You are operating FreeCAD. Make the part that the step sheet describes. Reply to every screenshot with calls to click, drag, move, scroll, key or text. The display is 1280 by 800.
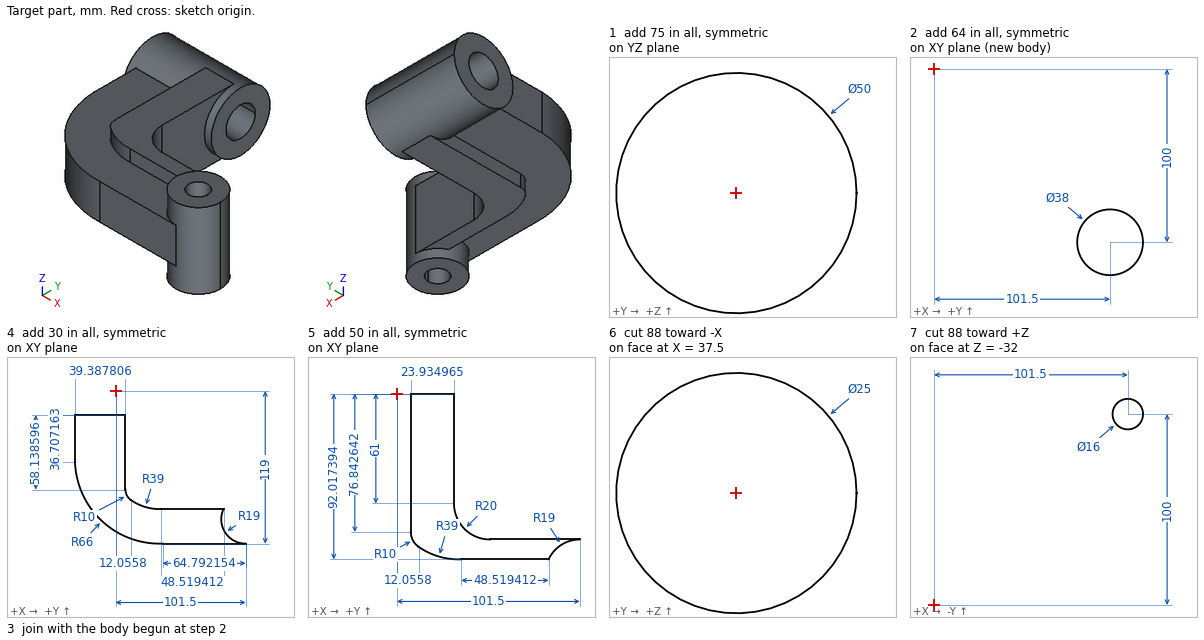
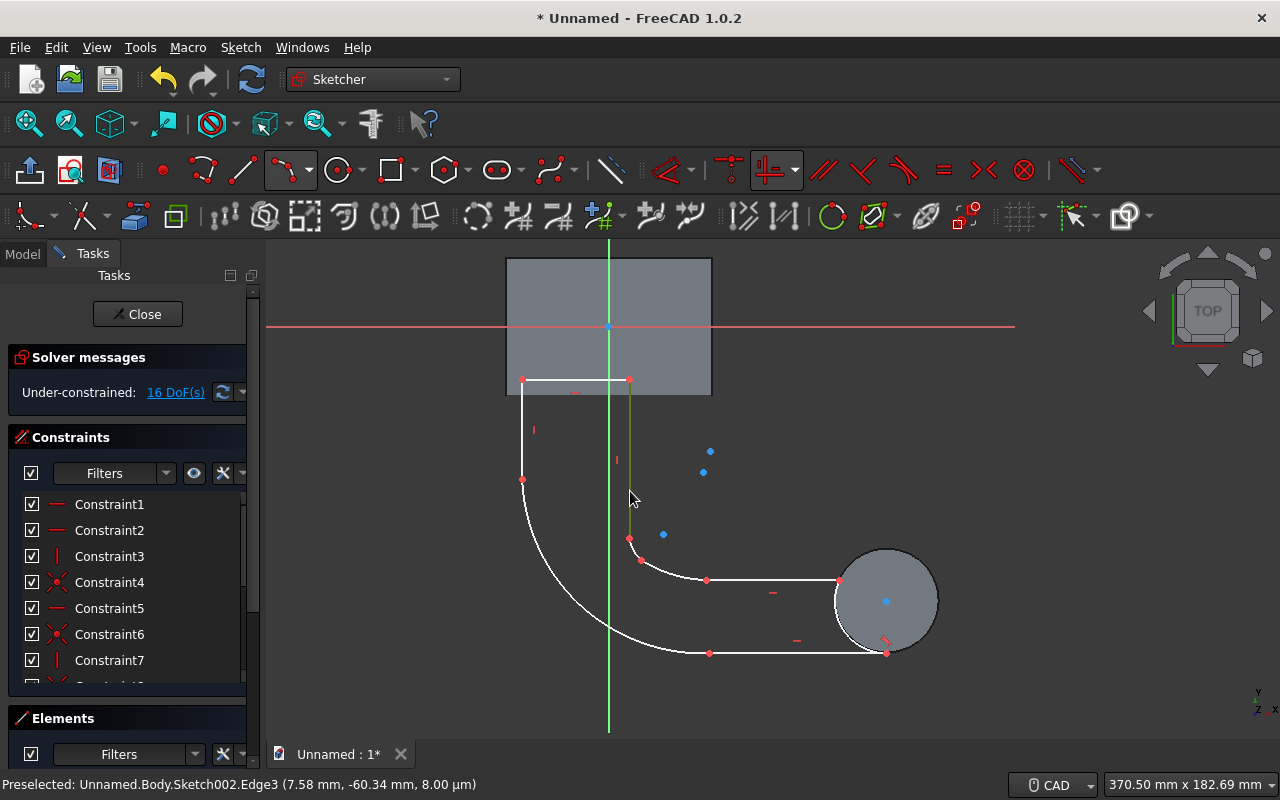
click(634, 551)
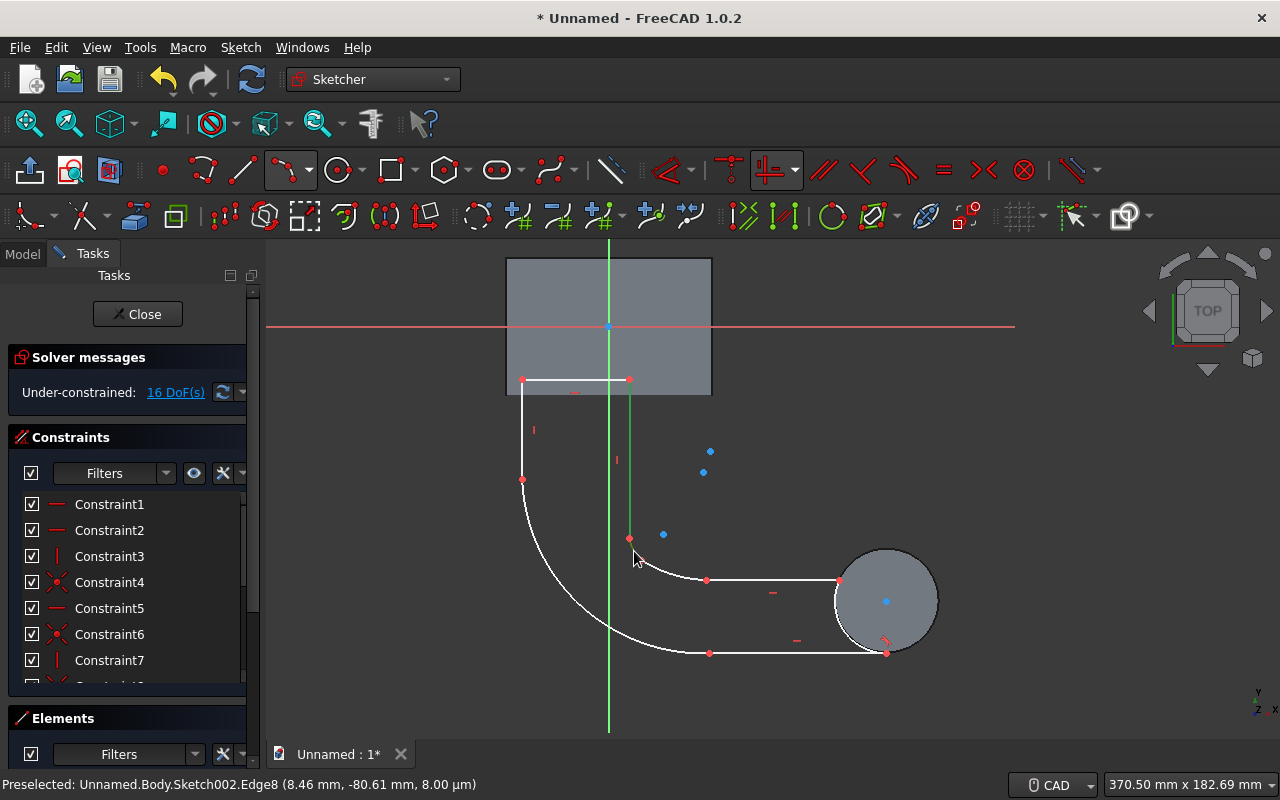
click(904, 170)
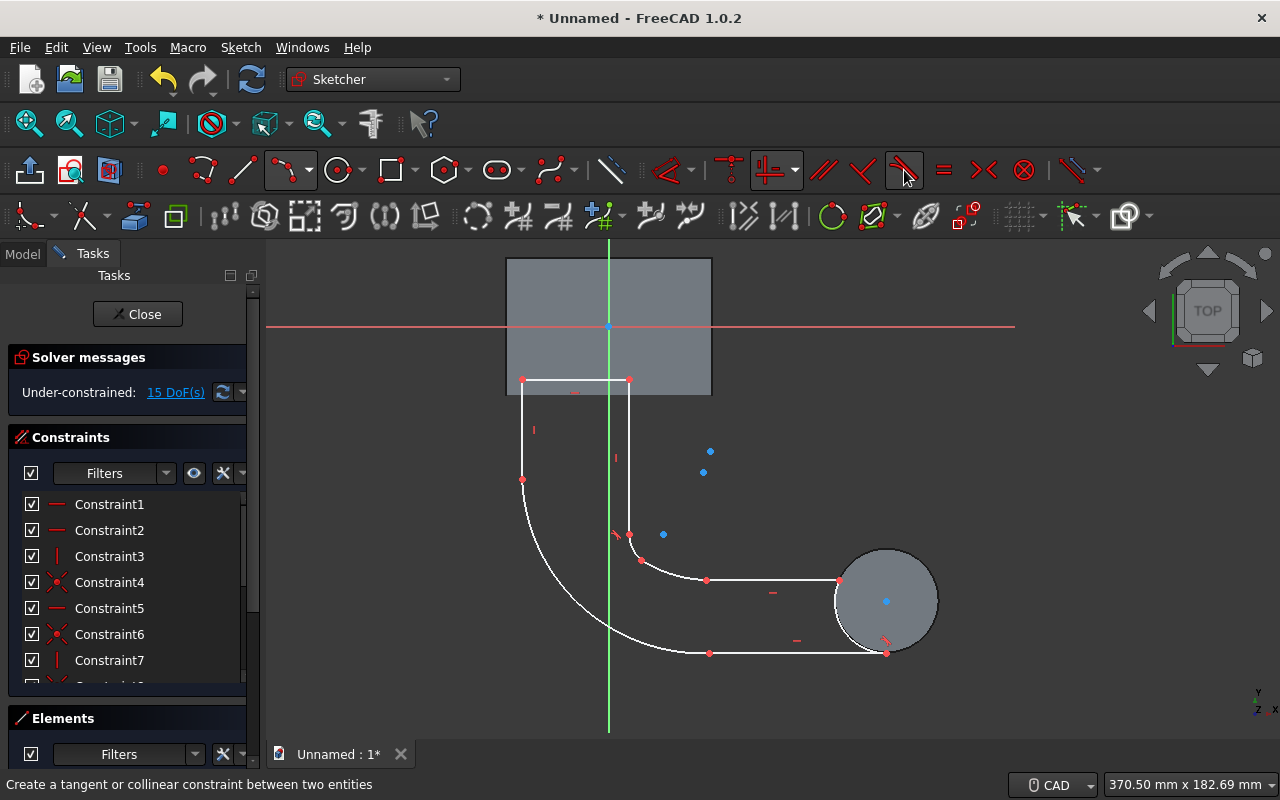
click(660, 570)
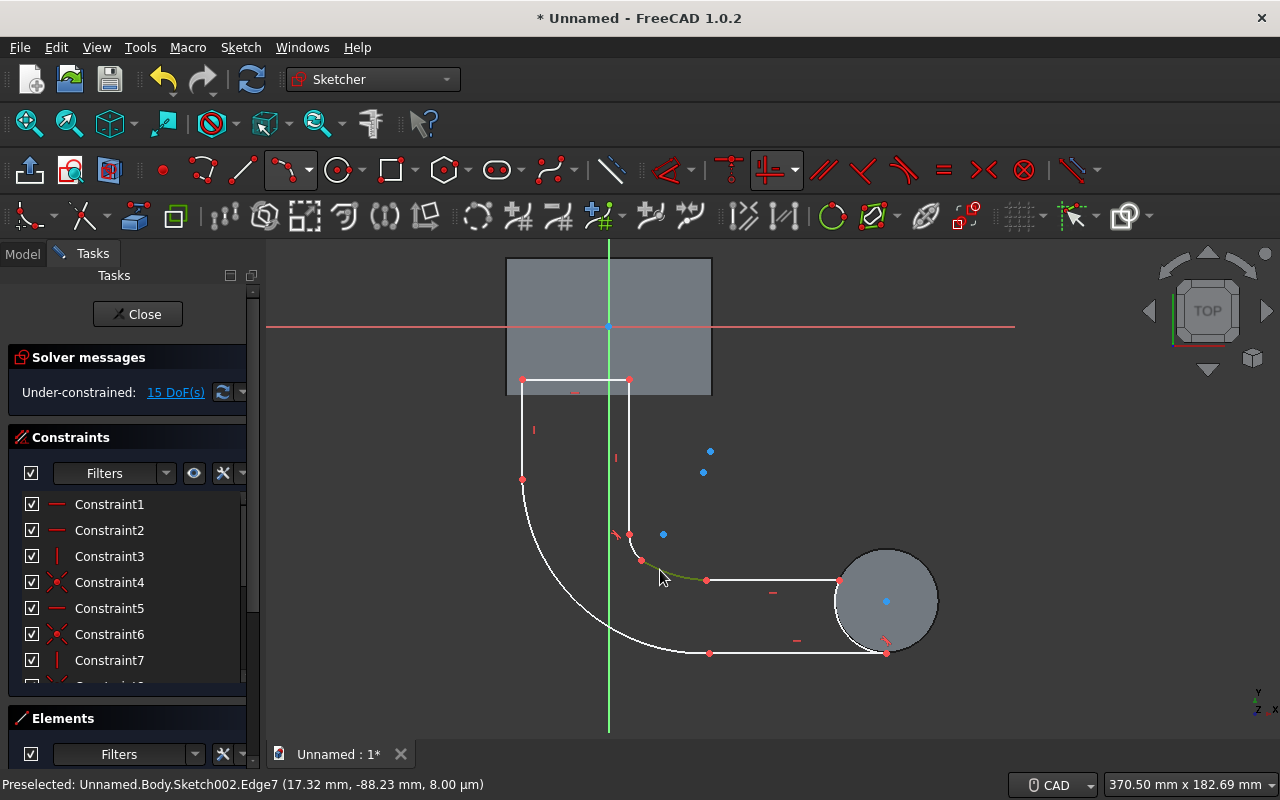
click(633, 549)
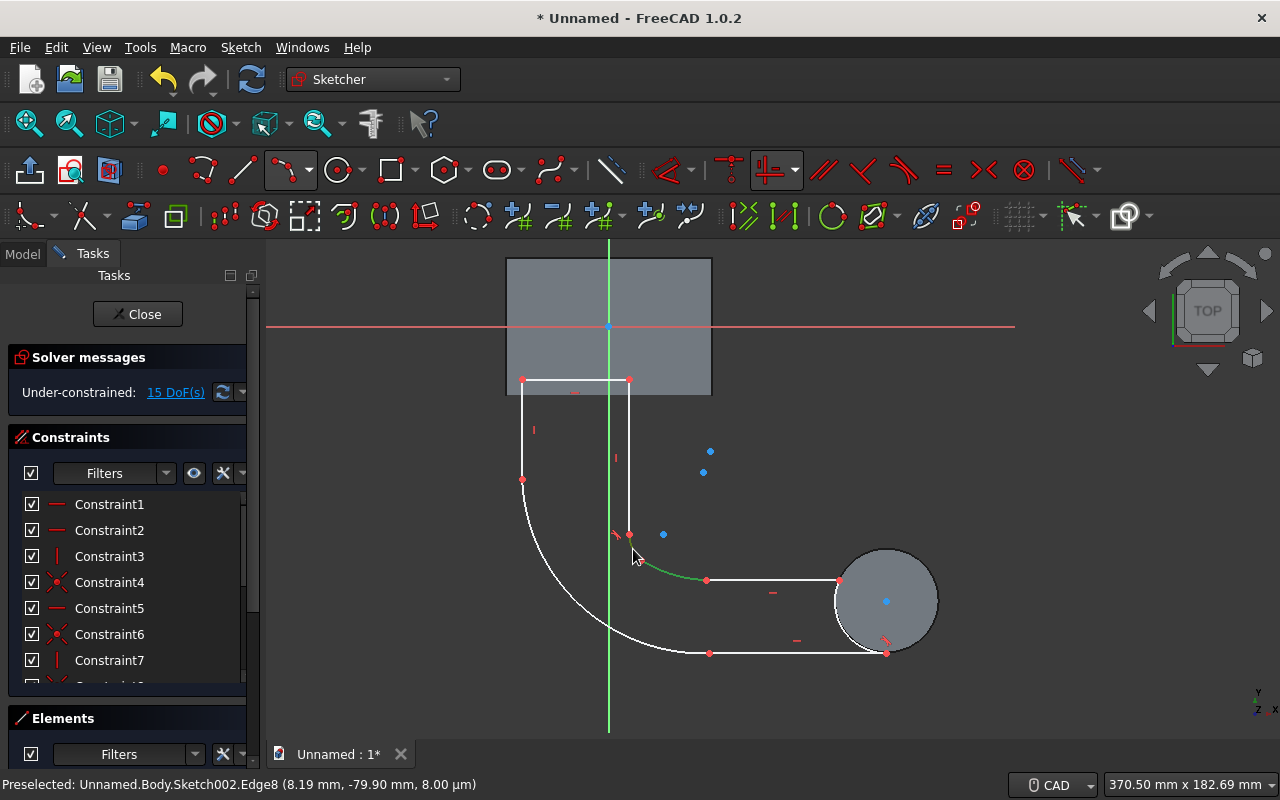
click(904, 170)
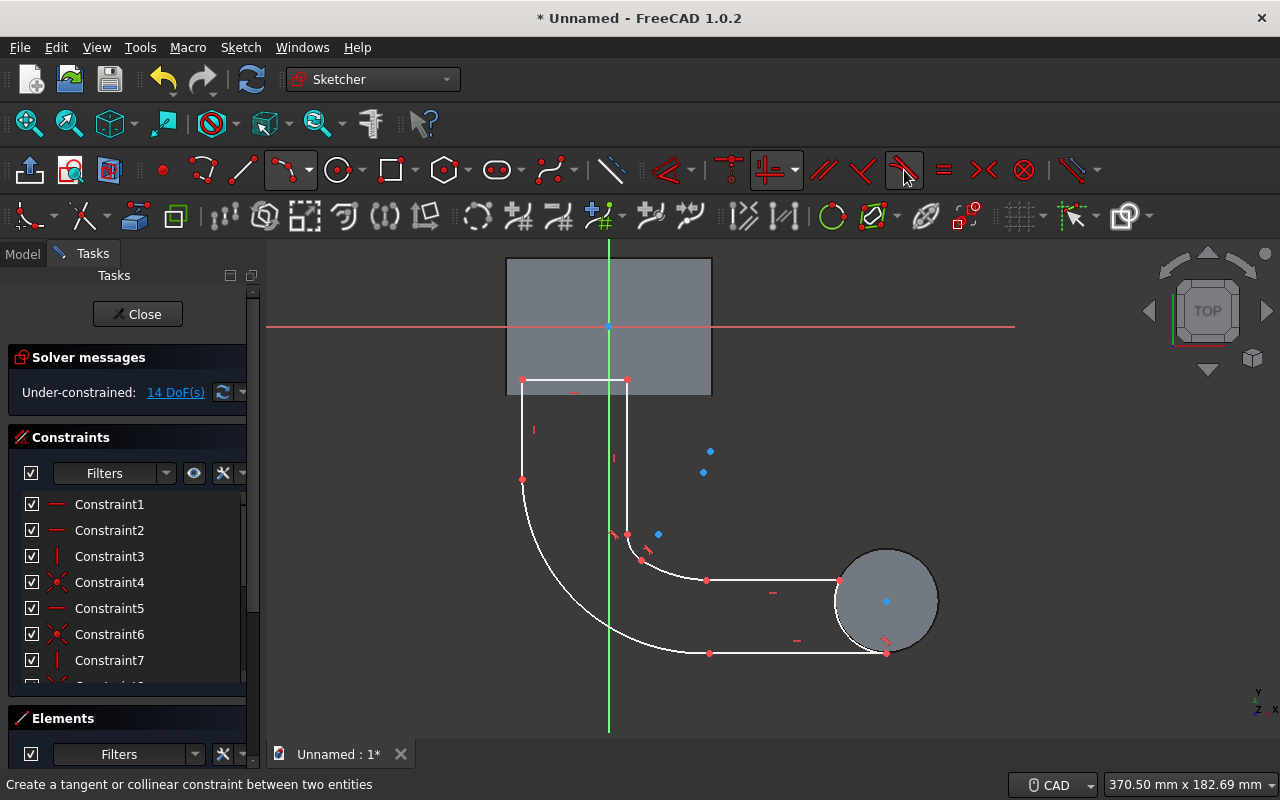
click(660, 570)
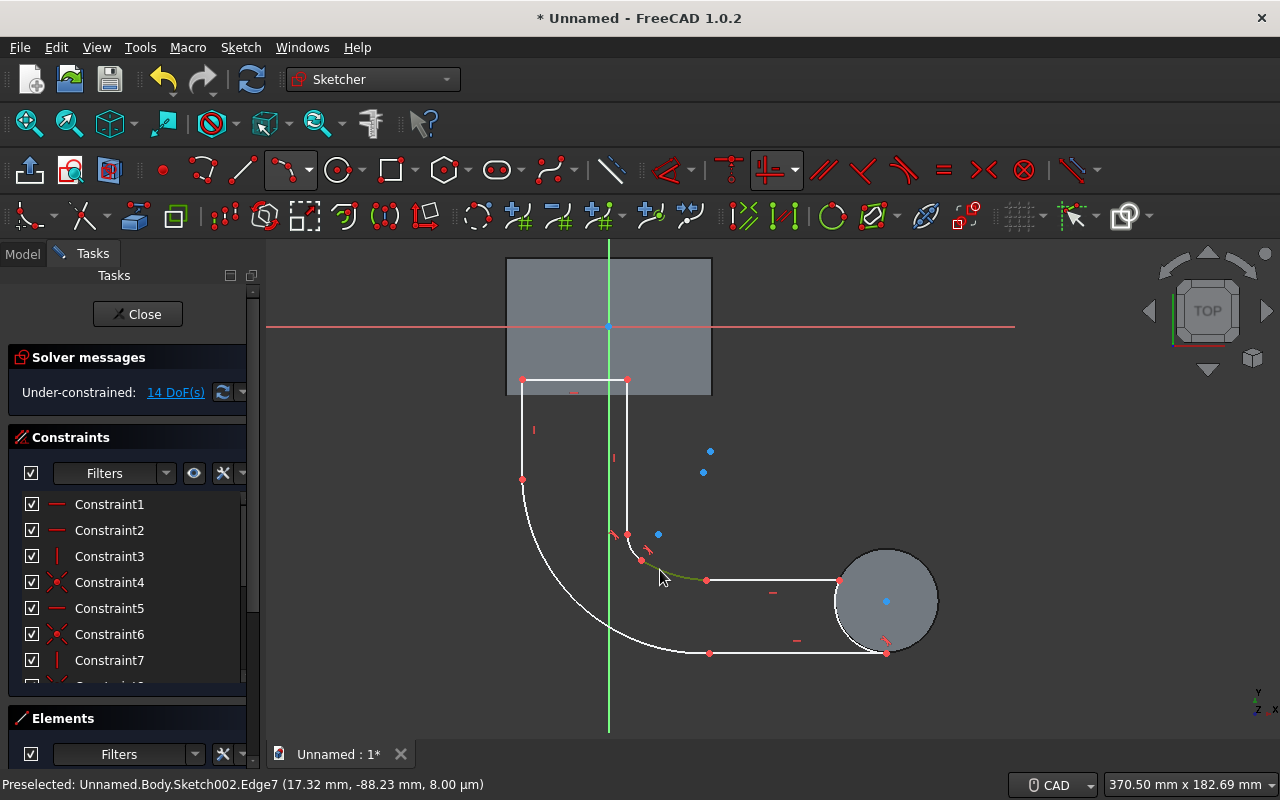
click(545, 561)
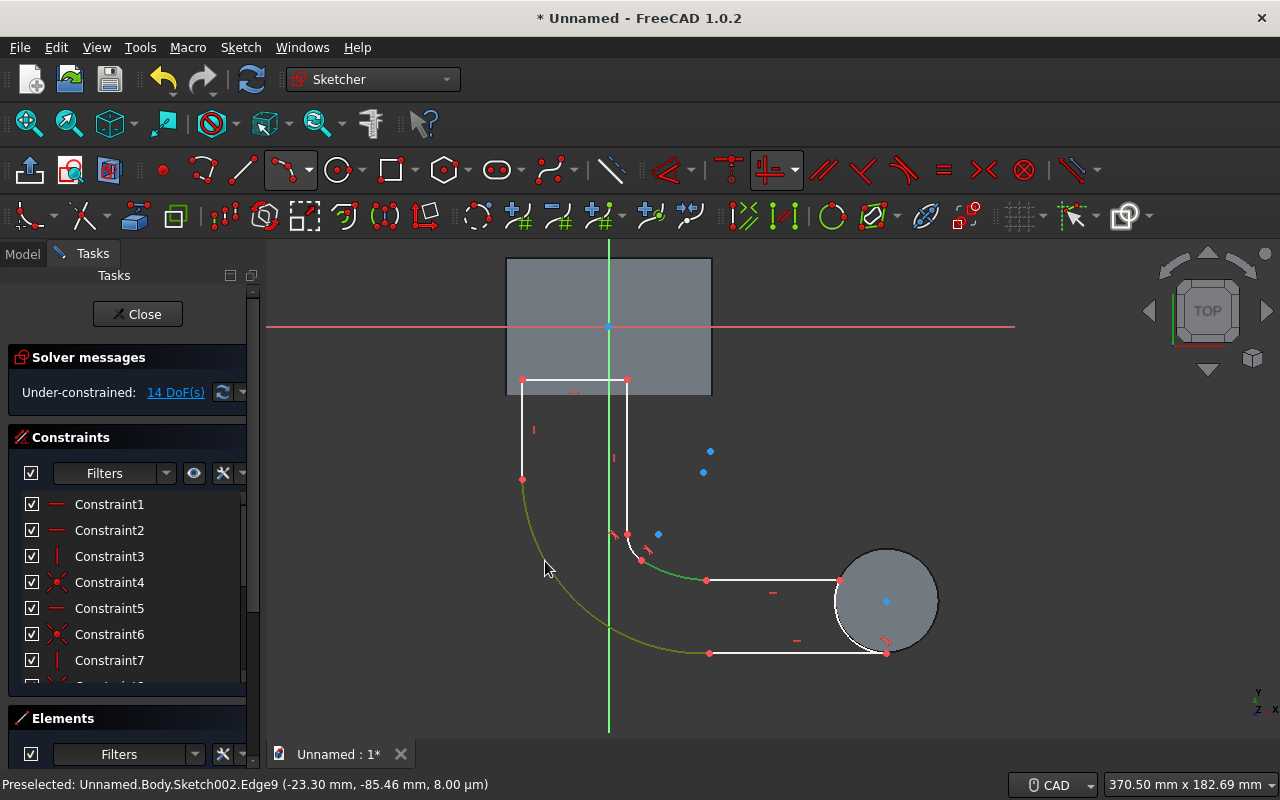
click(730, 170)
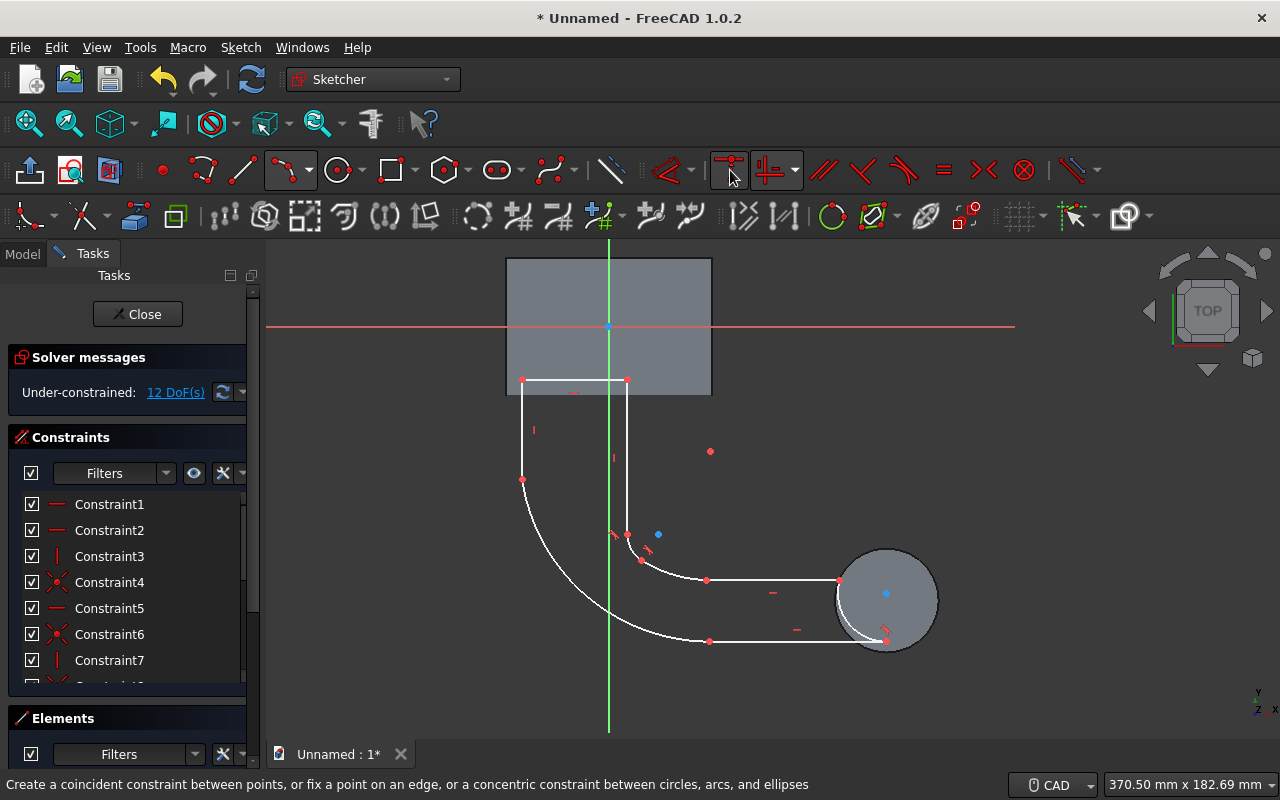
click(666, 170)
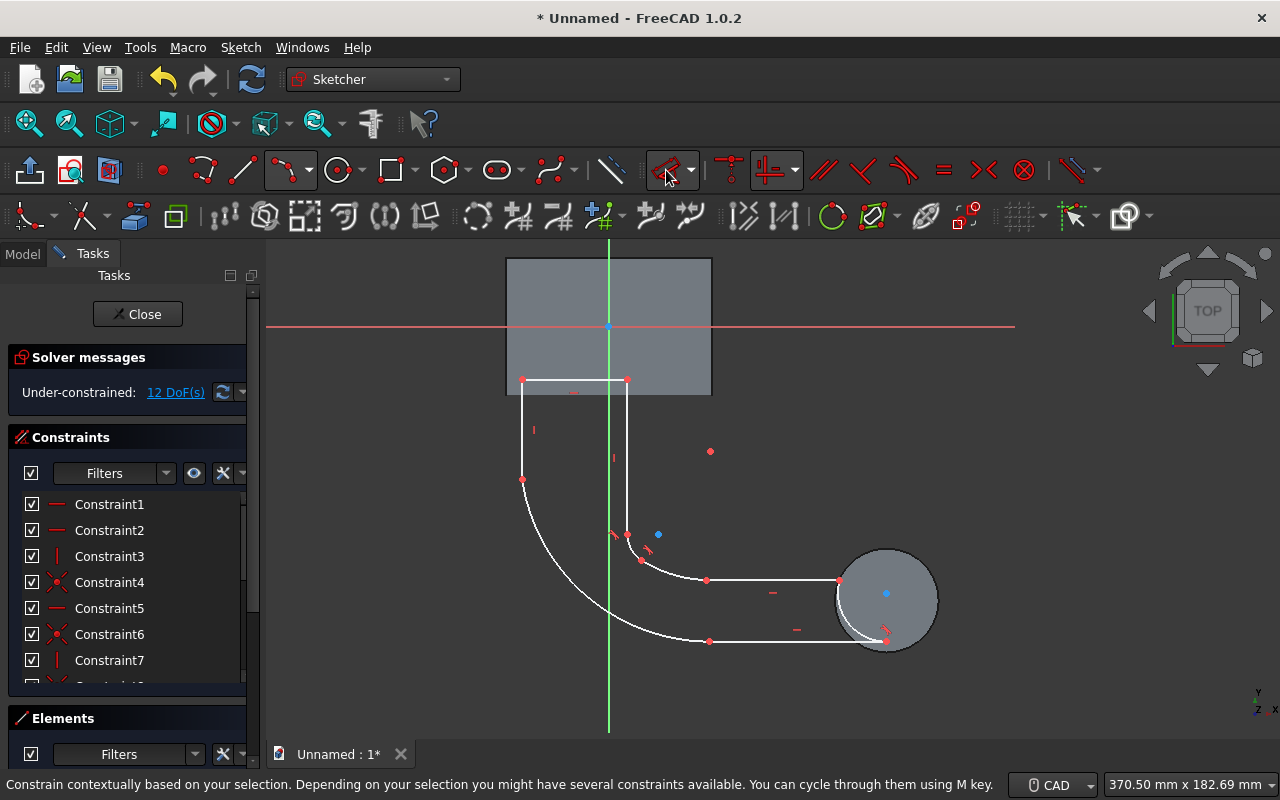
click(840, 607)
click(809, 616)